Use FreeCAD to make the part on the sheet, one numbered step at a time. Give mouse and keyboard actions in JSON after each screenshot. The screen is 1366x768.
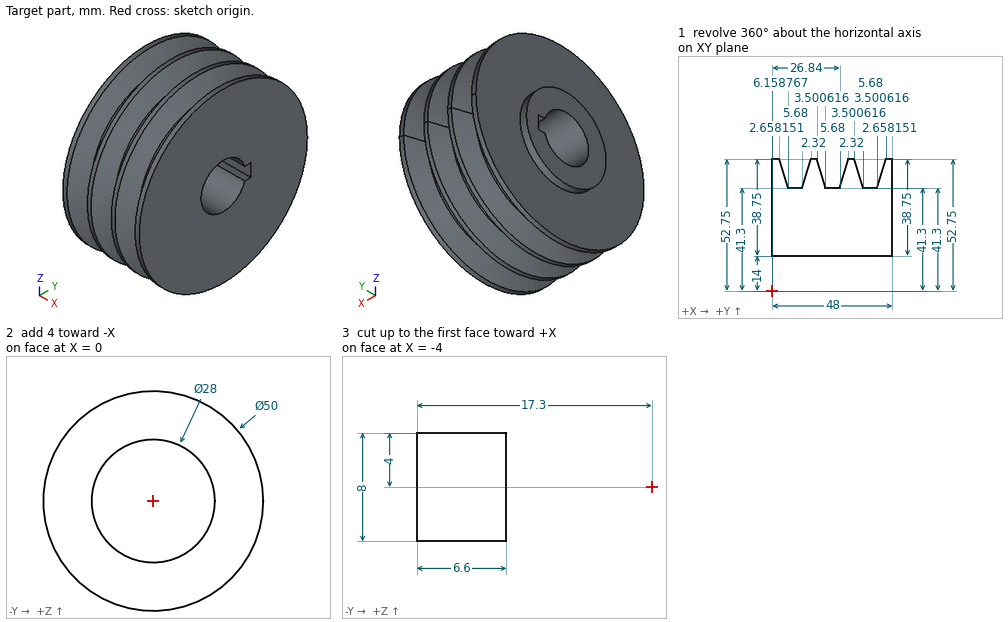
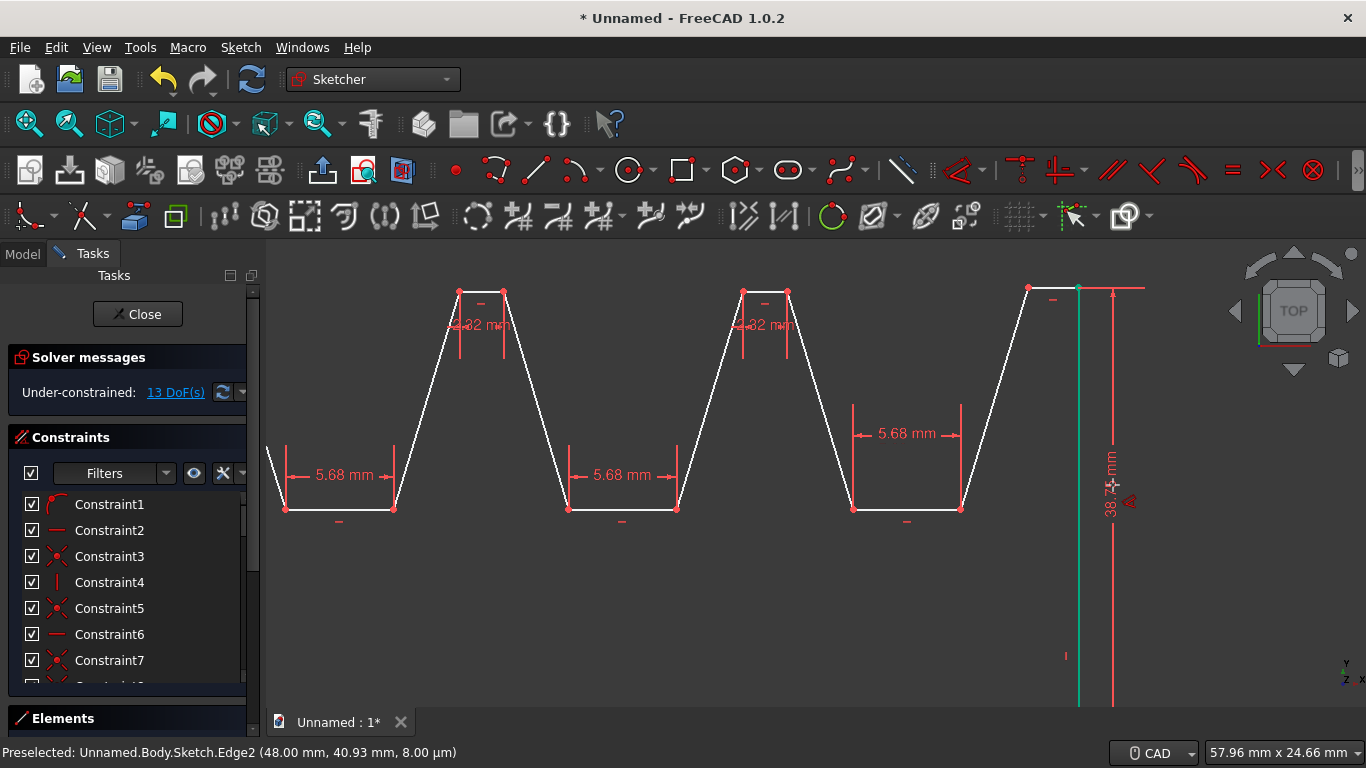
{"action": "scroll", "coordinate": [801, 337], "scroll_direction": "down", "scroll_amount": 6}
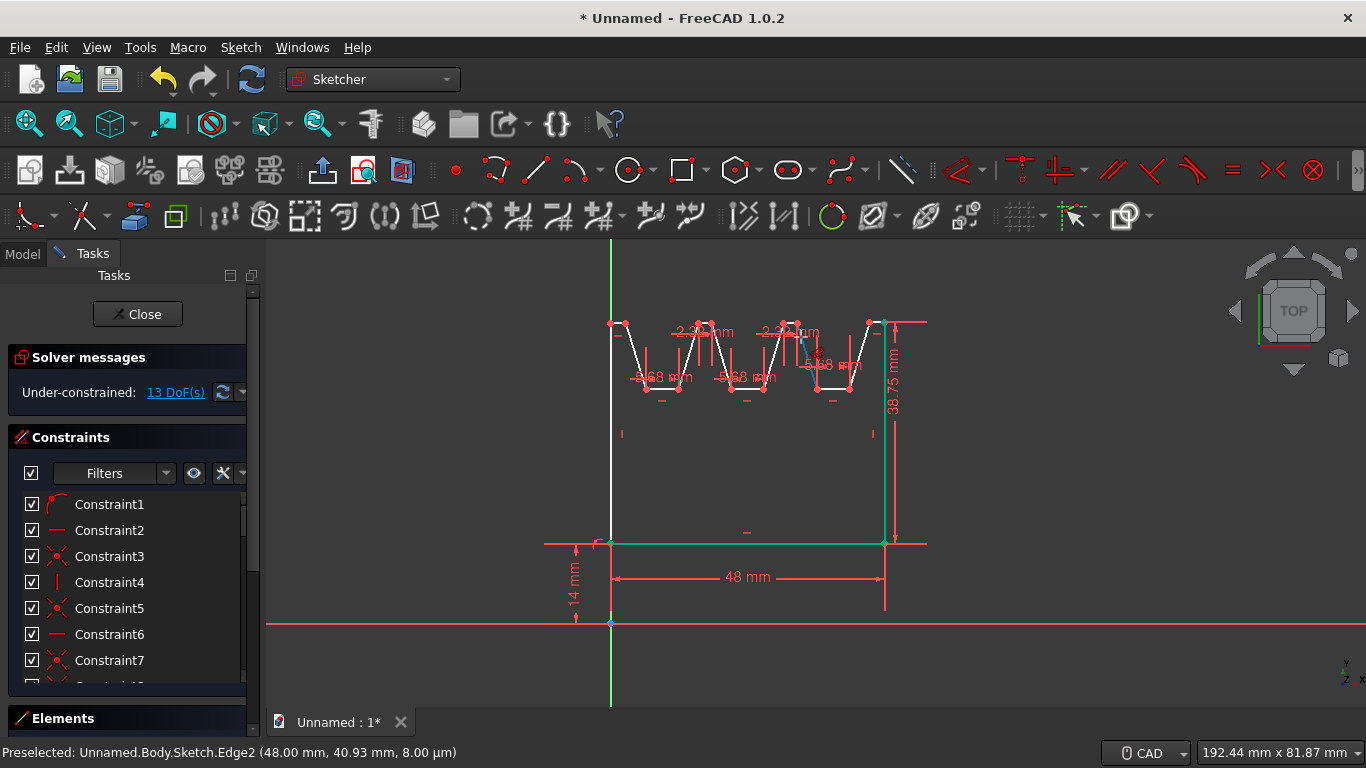
{"action": "left_click", "coordinate": [611, 390]}
{"action": "left_click", "coordinate": [577, 434]}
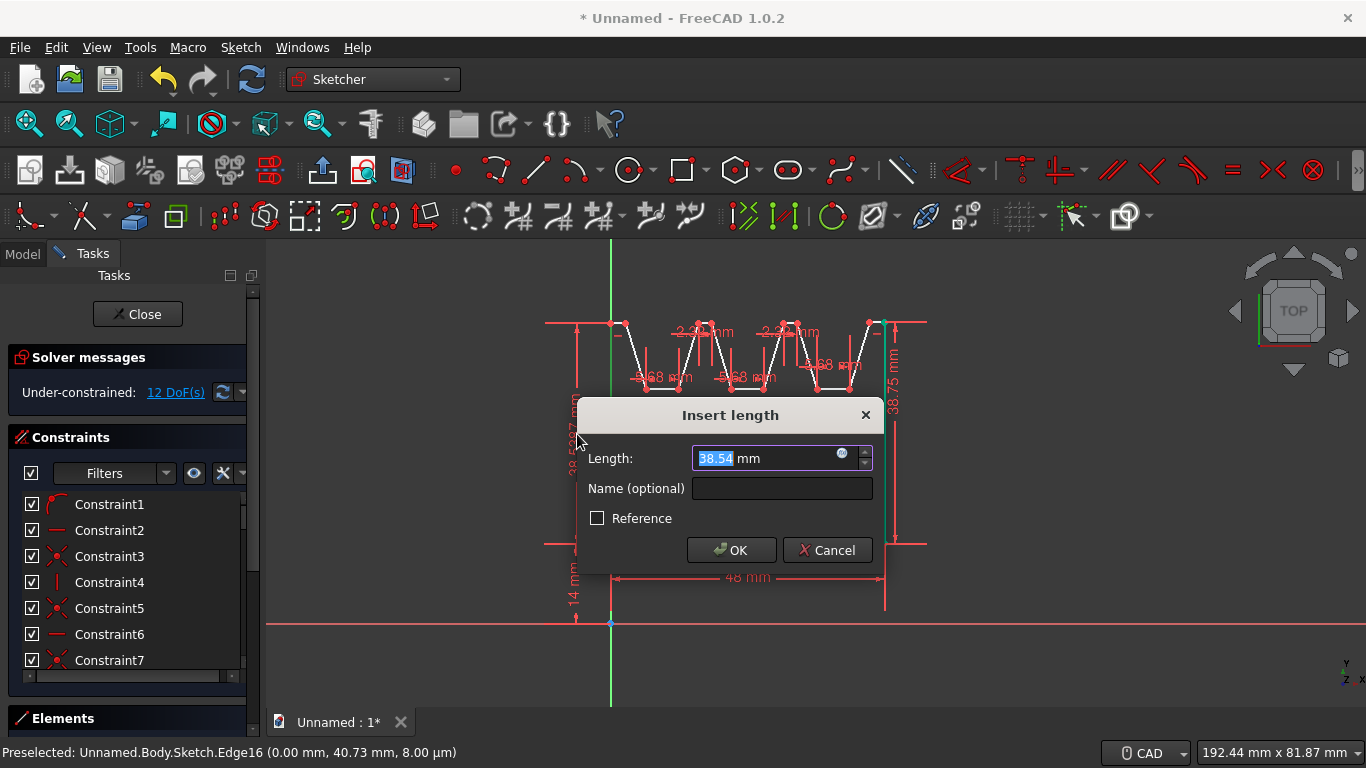
{"action": "type", "text": "38.75"}
{"action": "key", "text": "Return"}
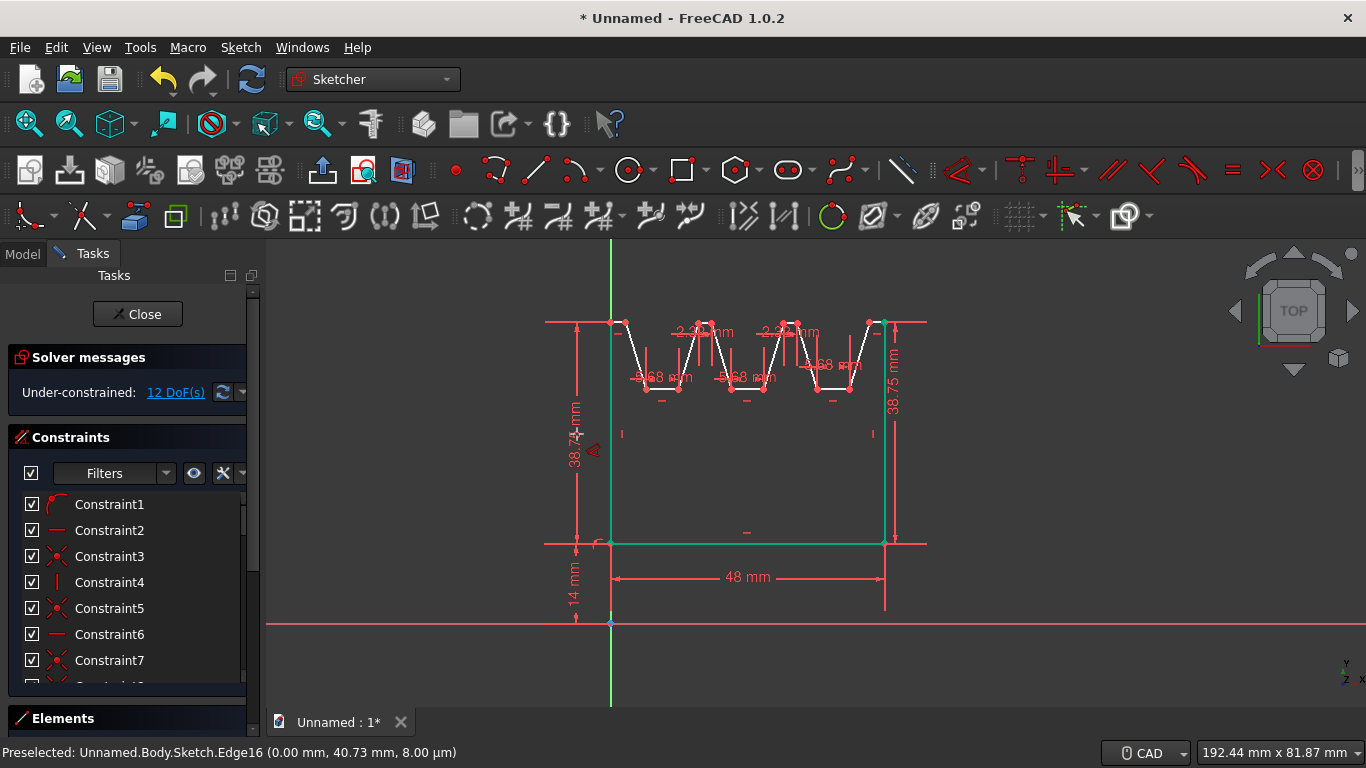
{"action": "left_click", "coordinate": [850, 389]}
{"action": "left_click", "coordinate": [577, 506]}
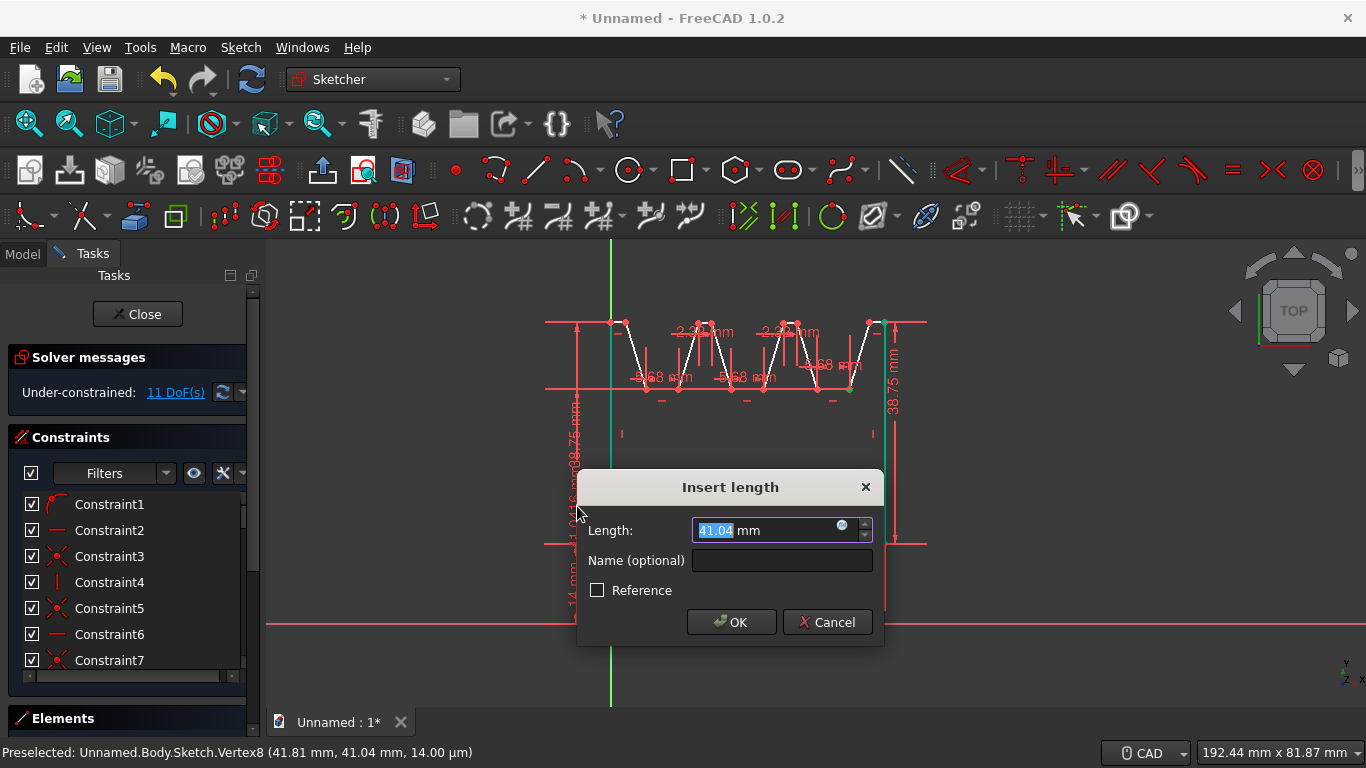
{"action": "type", "text": "41.3"}
{"action": "key", "text": "Return"}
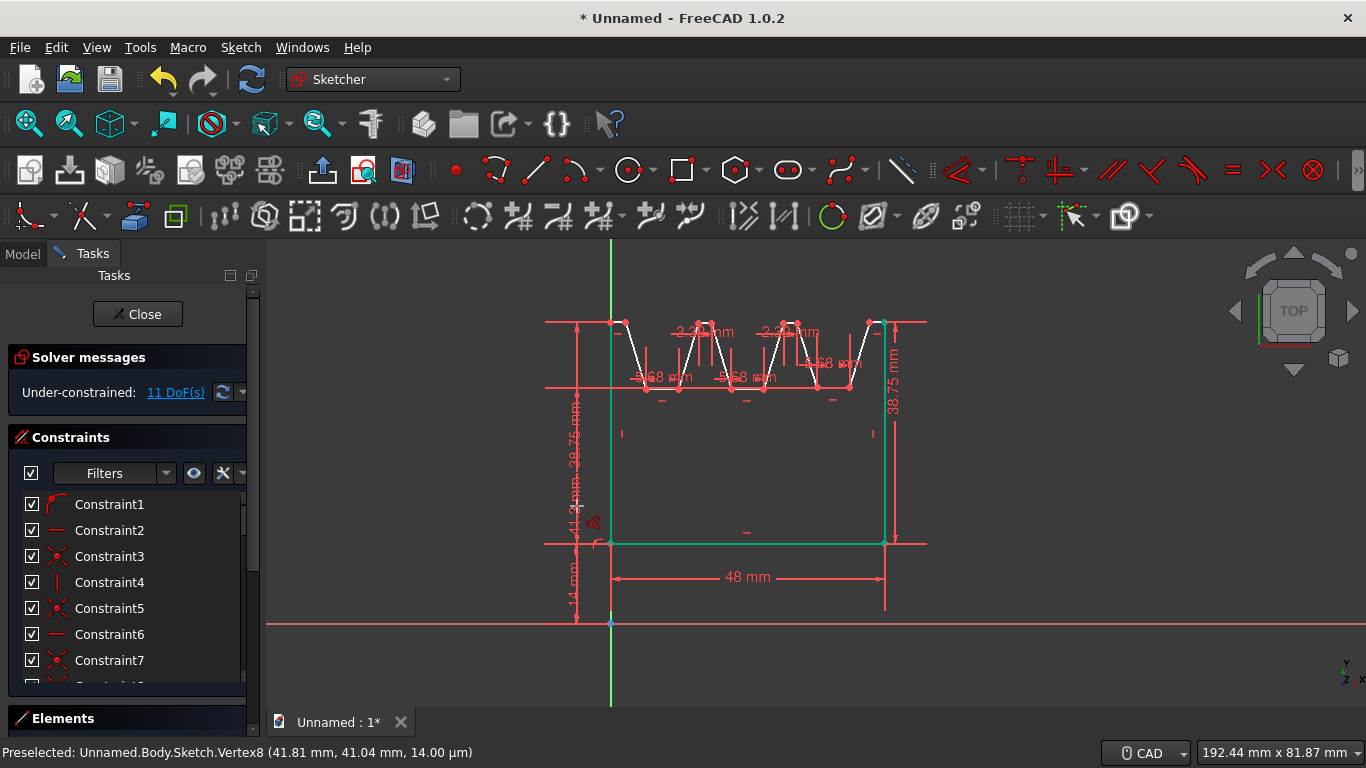
{"action": "left_click", "coordinate": [764, 389]}
{"action": "left_click", "coordinate": [577, 560]}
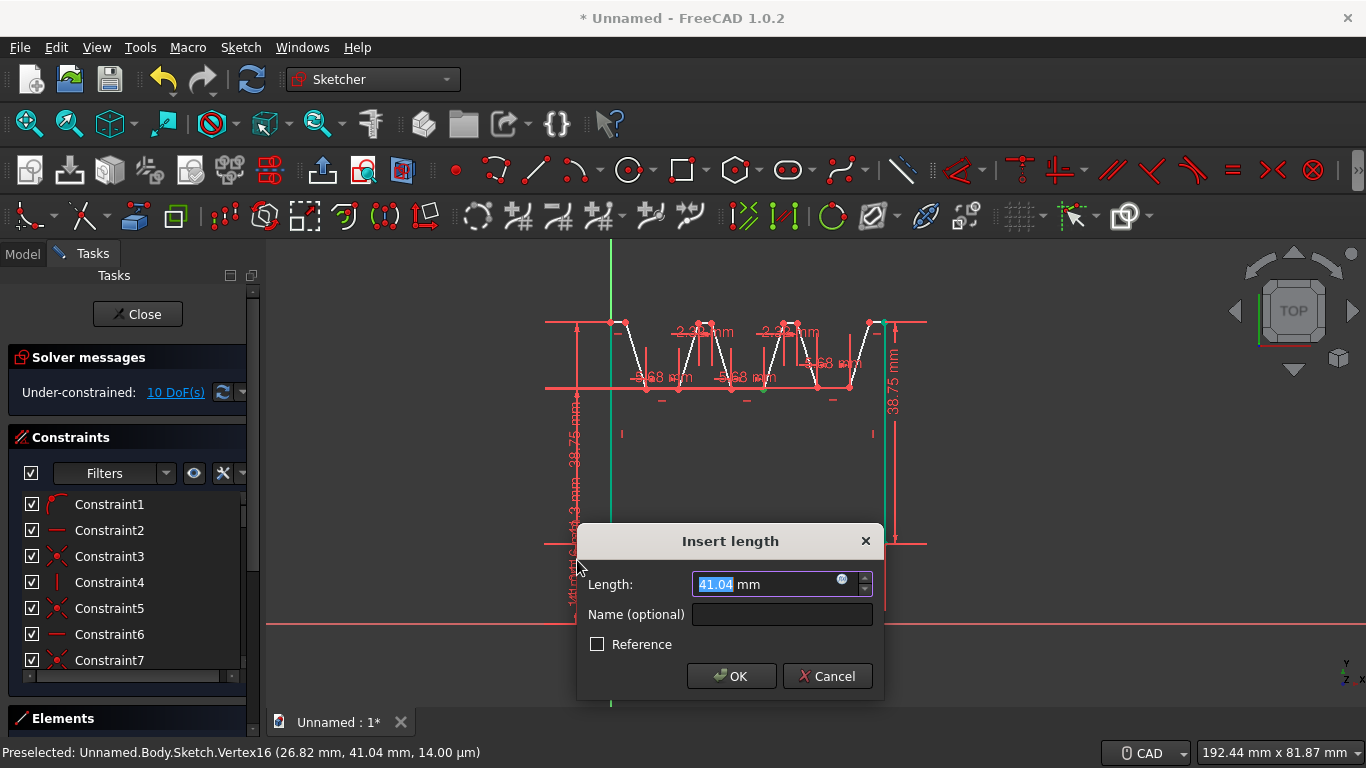
{"action": "type", "text": "41.3"}
{"action": "key", "text": "Return"}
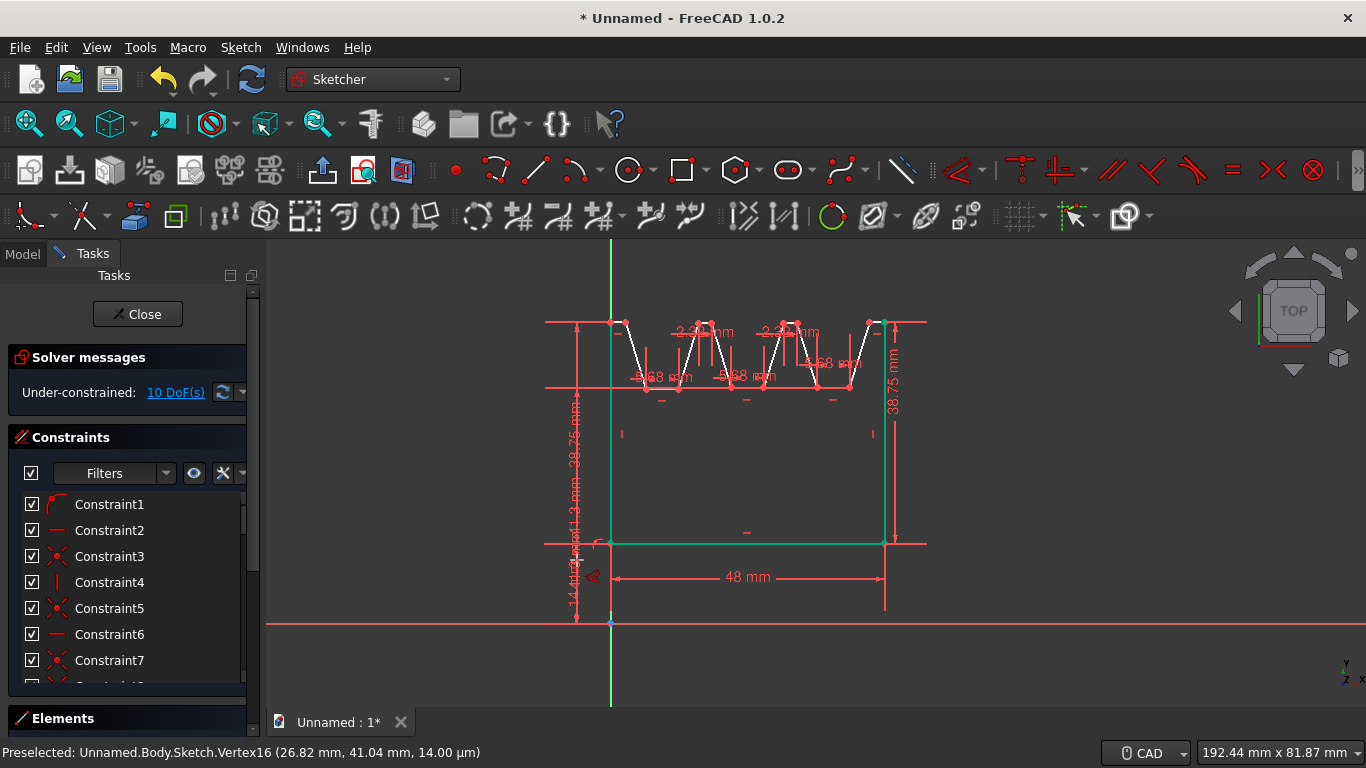
{"action": "left_click", "coordinate": [679, 389]}
{"action": "left_click", "coordinate": [713, 506]}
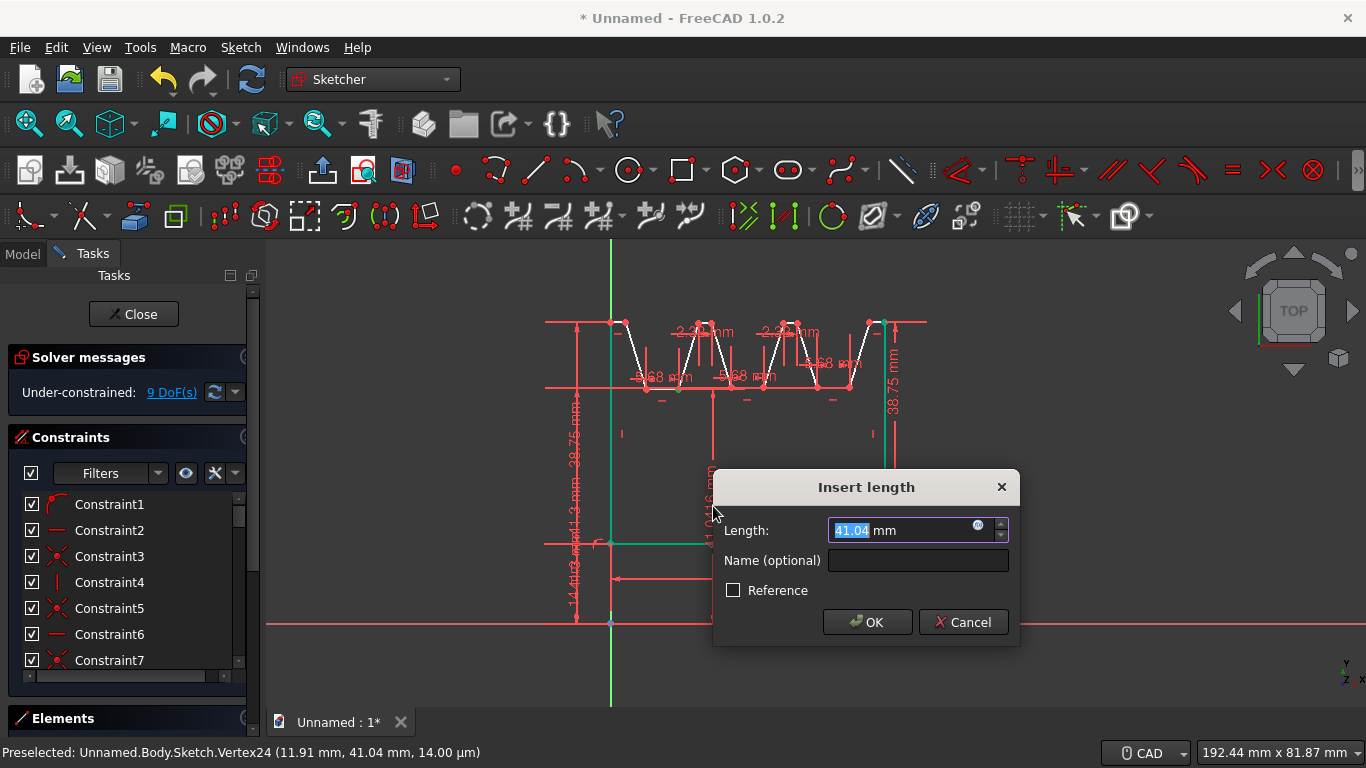
{"action": "type", "text": "41.3"}
{"action": "key", "text": "Return"}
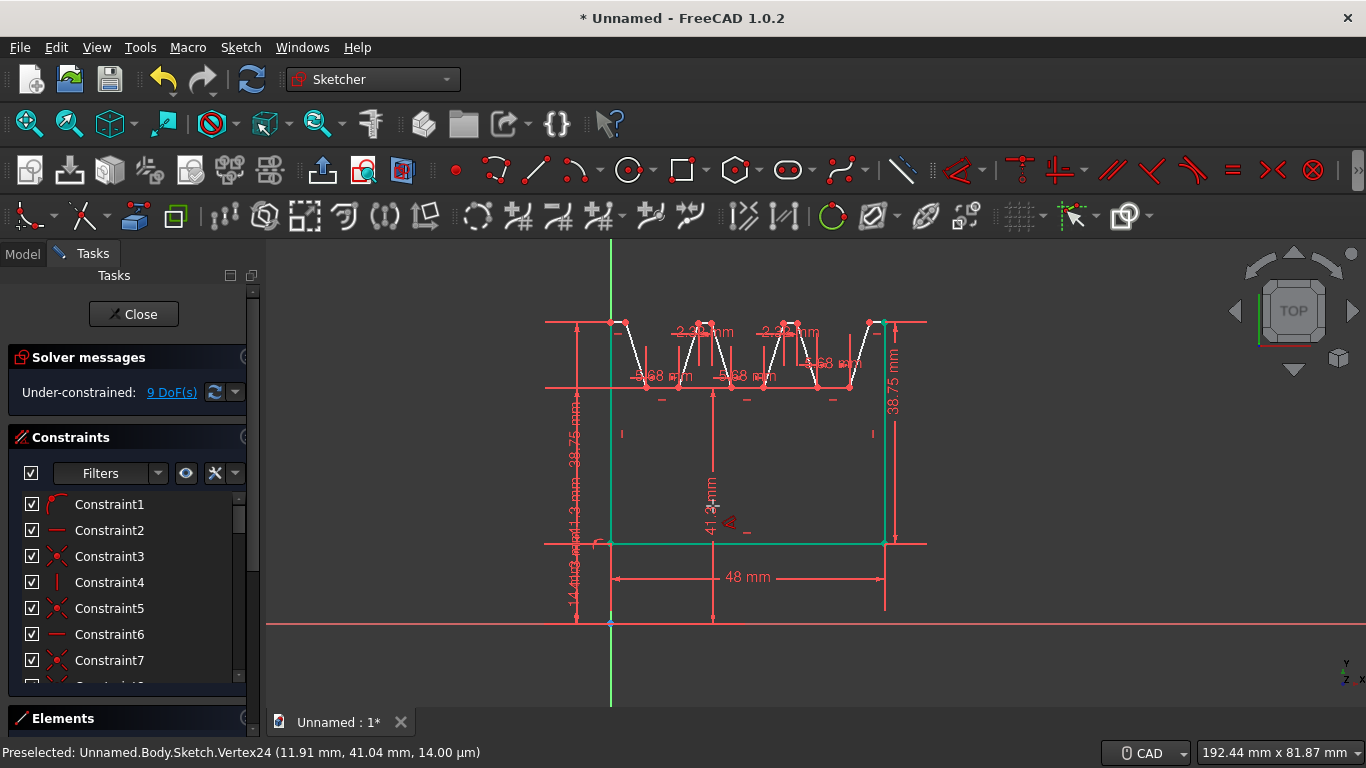
{"action": "left_click", "coordinate": [797, 323]}
{"action": "left_click", "coordinate": [577, 474]}